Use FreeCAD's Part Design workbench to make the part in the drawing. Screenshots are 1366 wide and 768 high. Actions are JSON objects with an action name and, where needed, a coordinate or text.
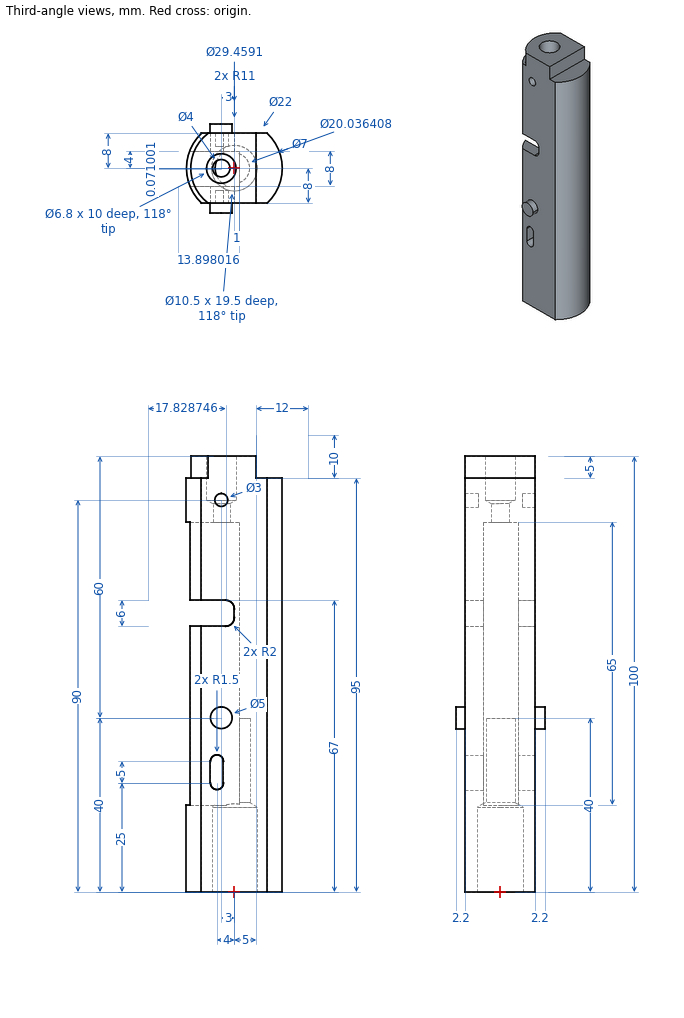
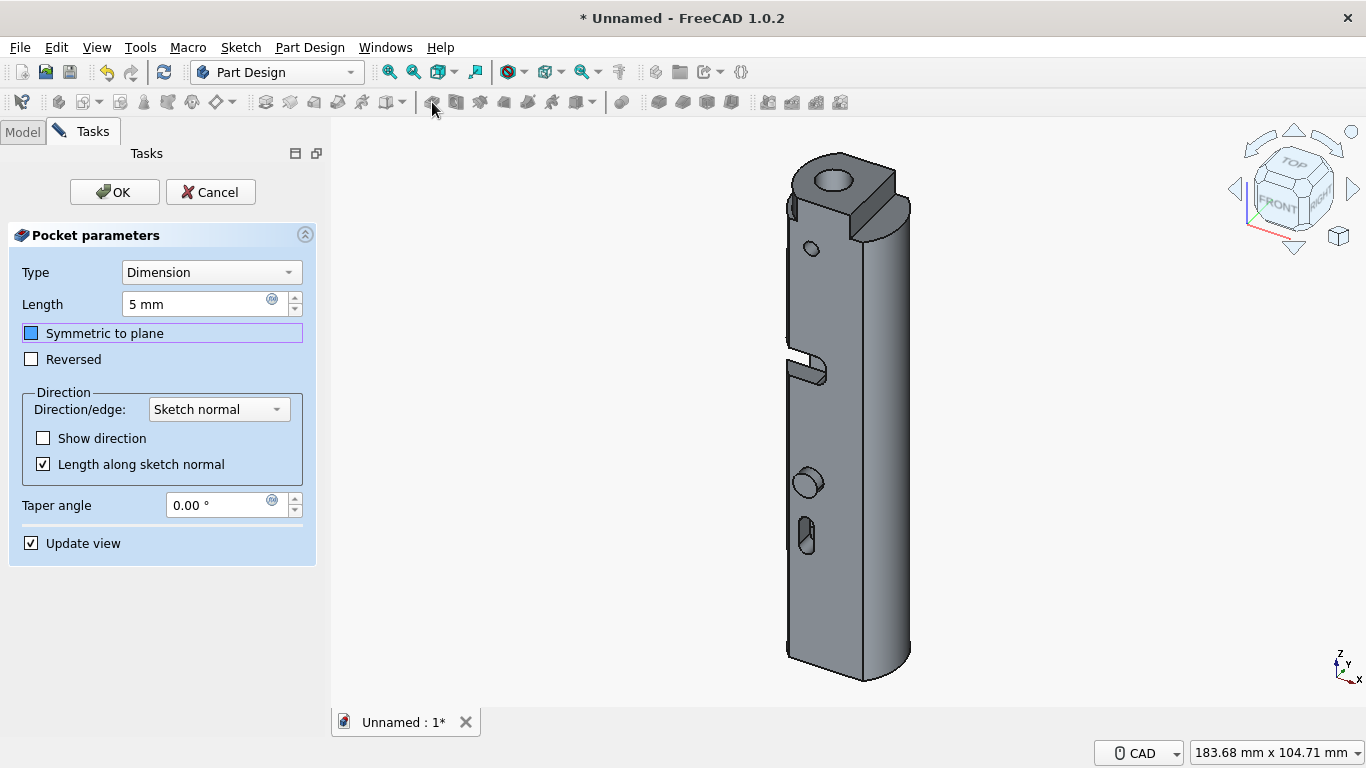
{"action": "left_click", "coordinate": [115, 192]}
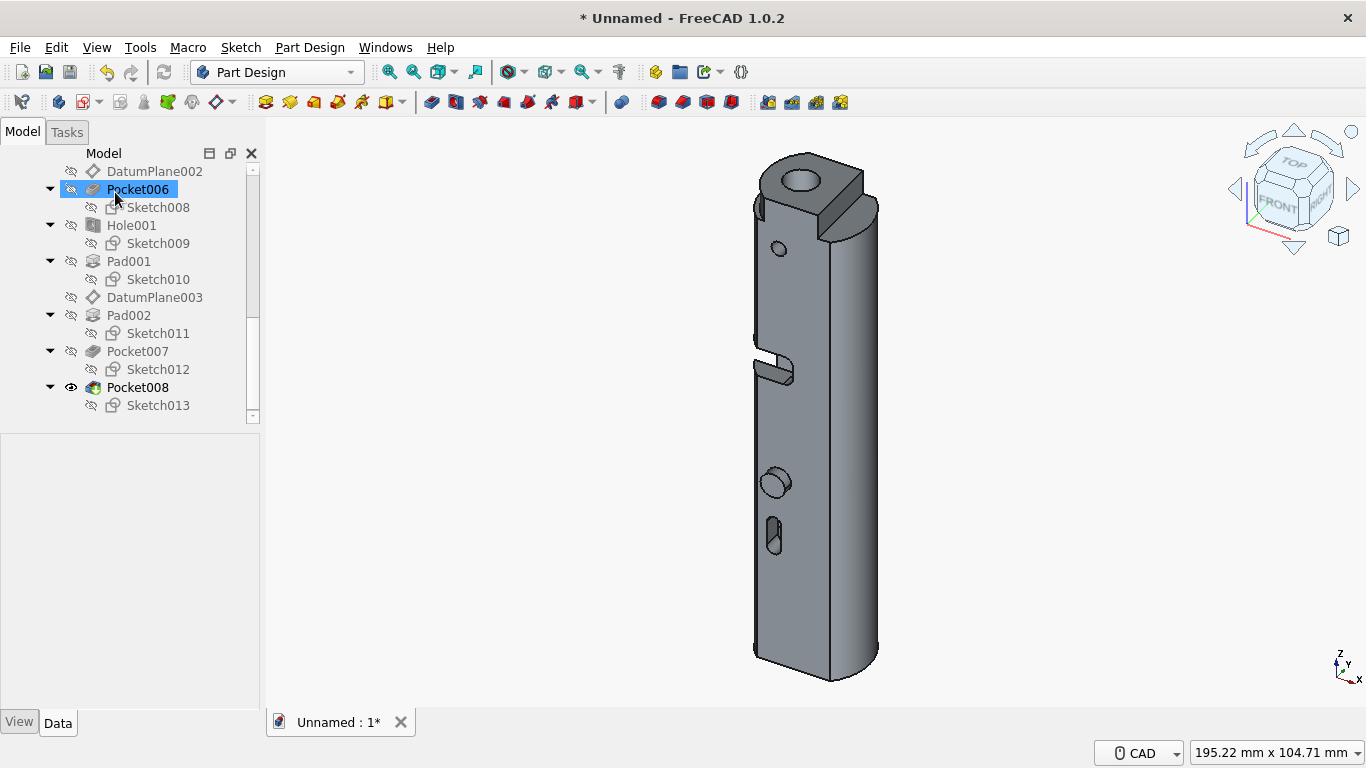
{"action": "key", "text": "0"}